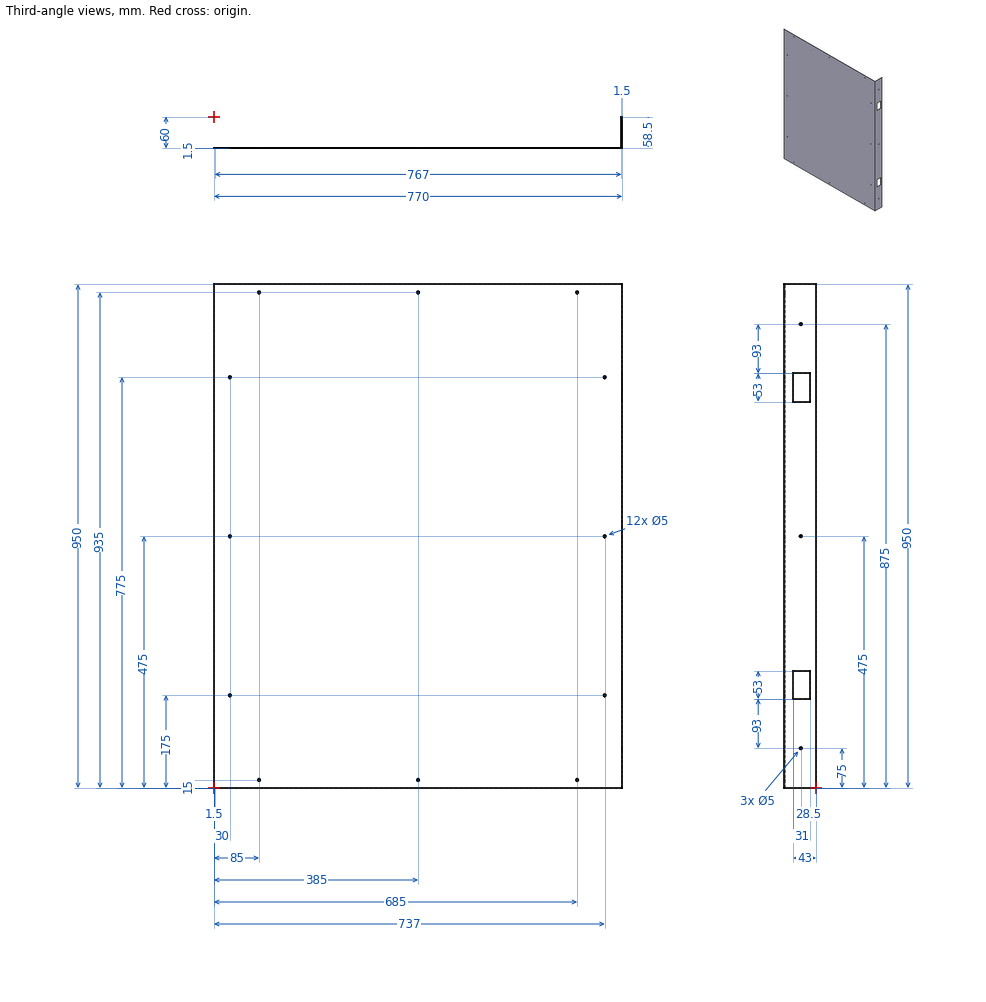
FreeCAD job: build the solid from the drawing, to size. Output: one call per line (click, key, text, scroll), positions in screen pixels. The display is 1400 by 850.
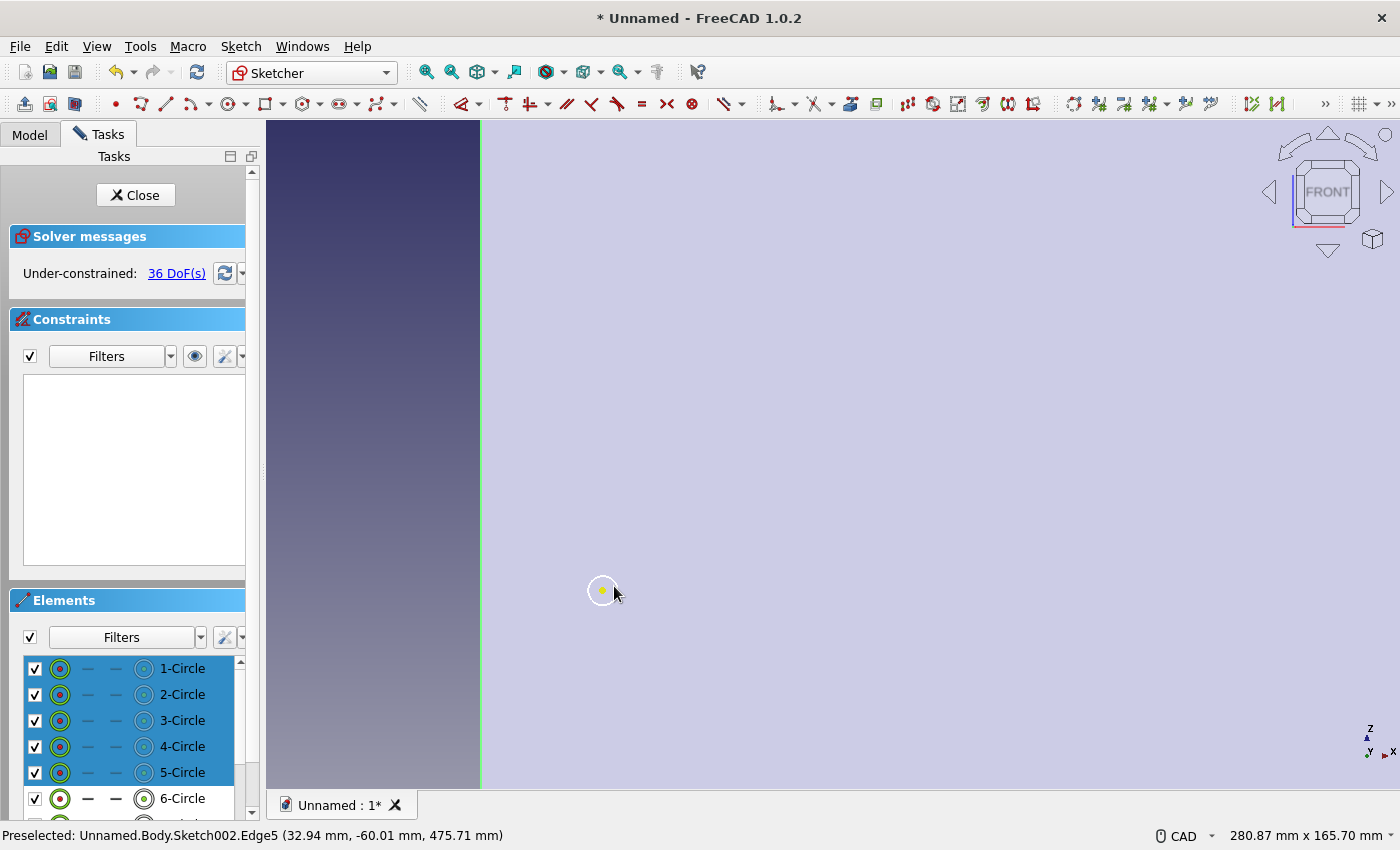
click(613, 580)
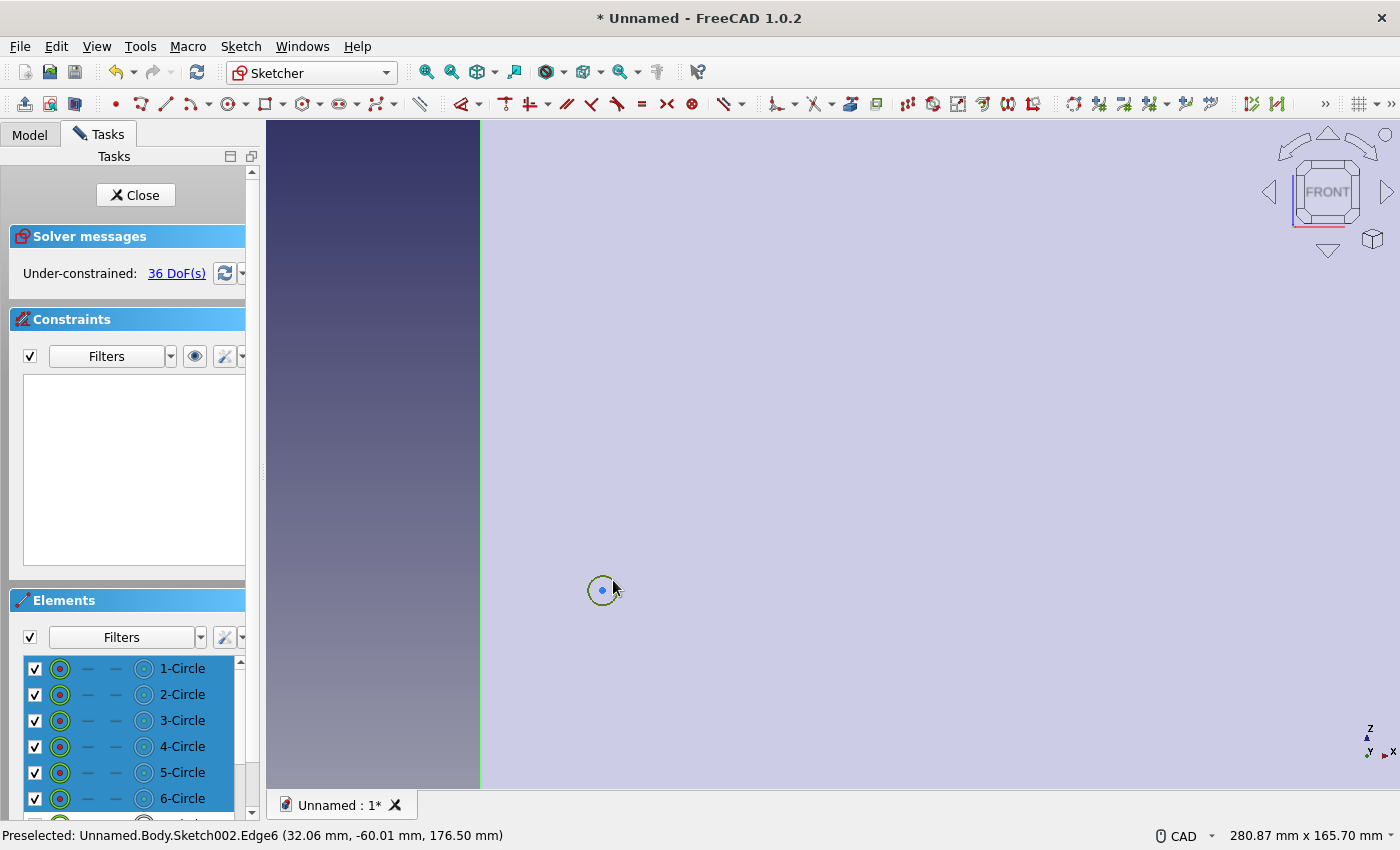
scroll(614, 586, down, 11)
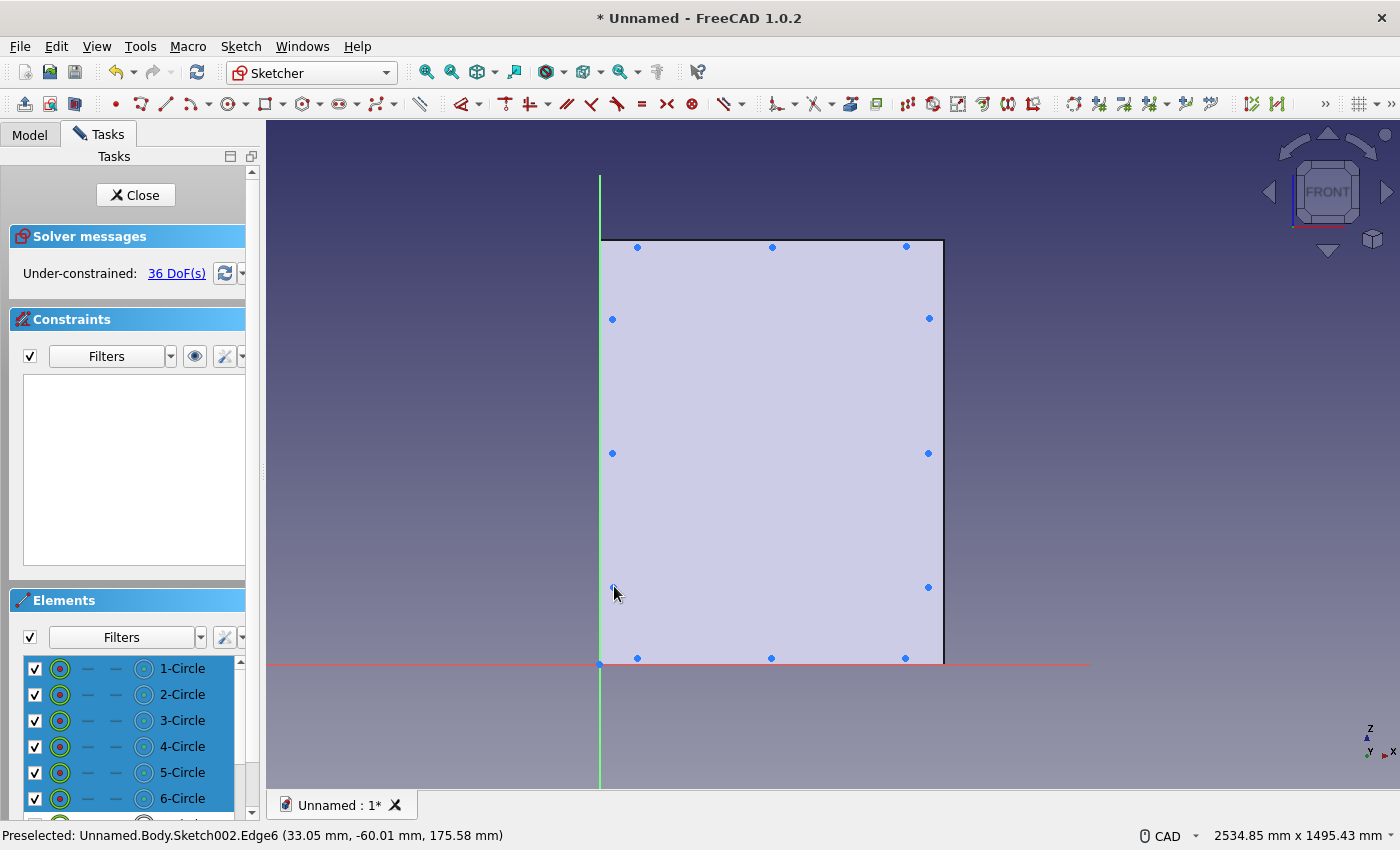
scroll(773, 246, up, 12)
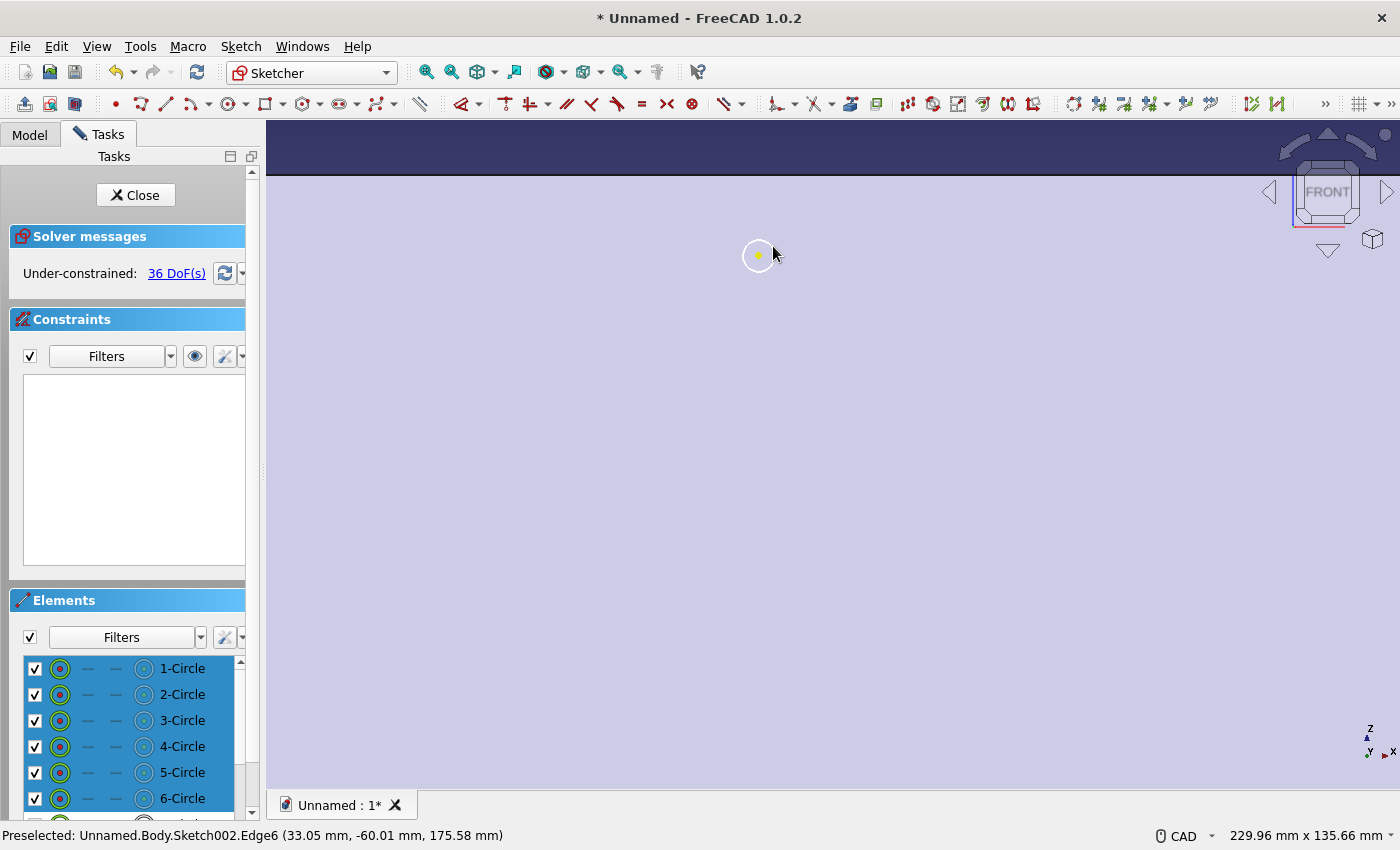
click(770, 245)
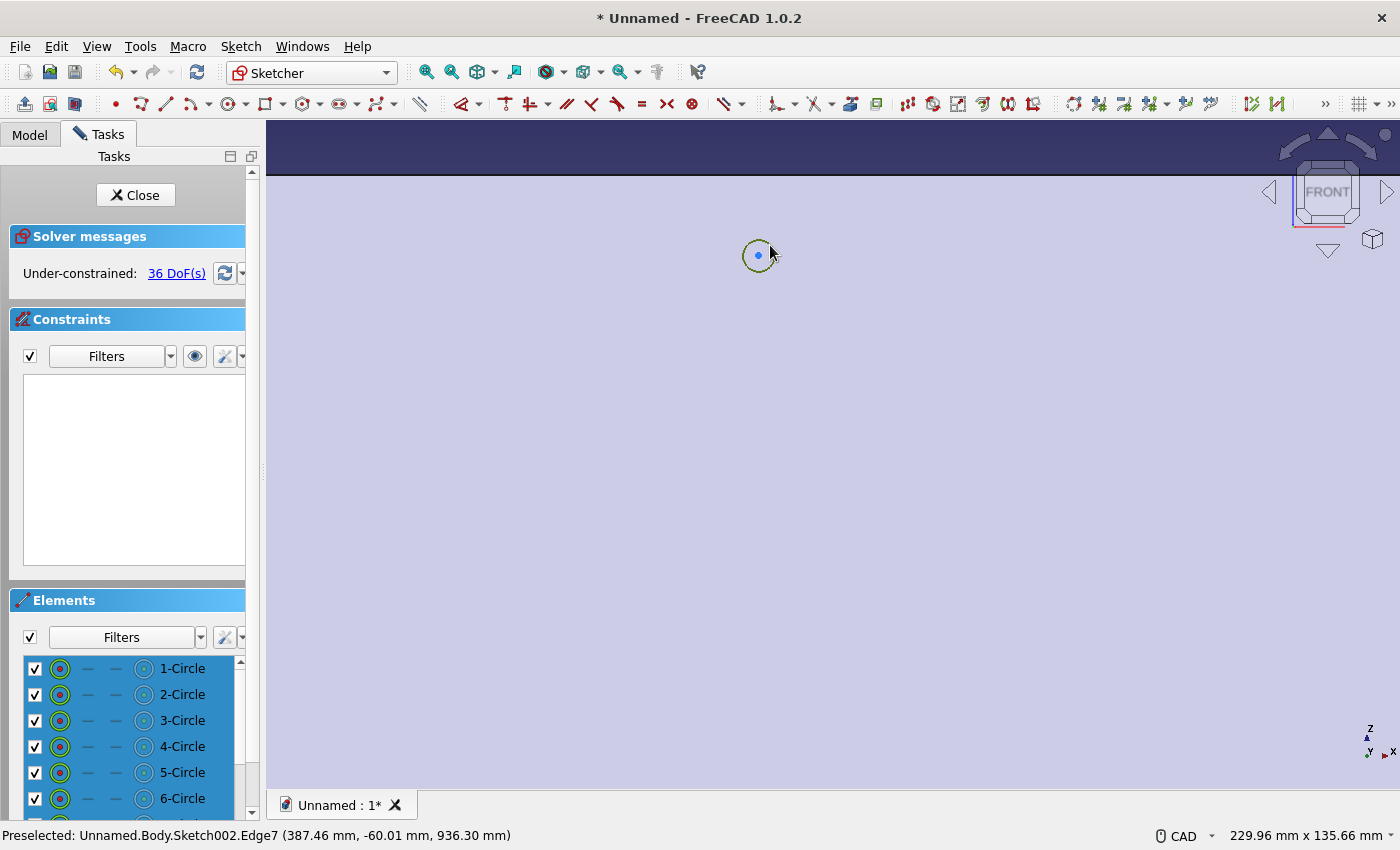
scroll(773, 246, down, 12)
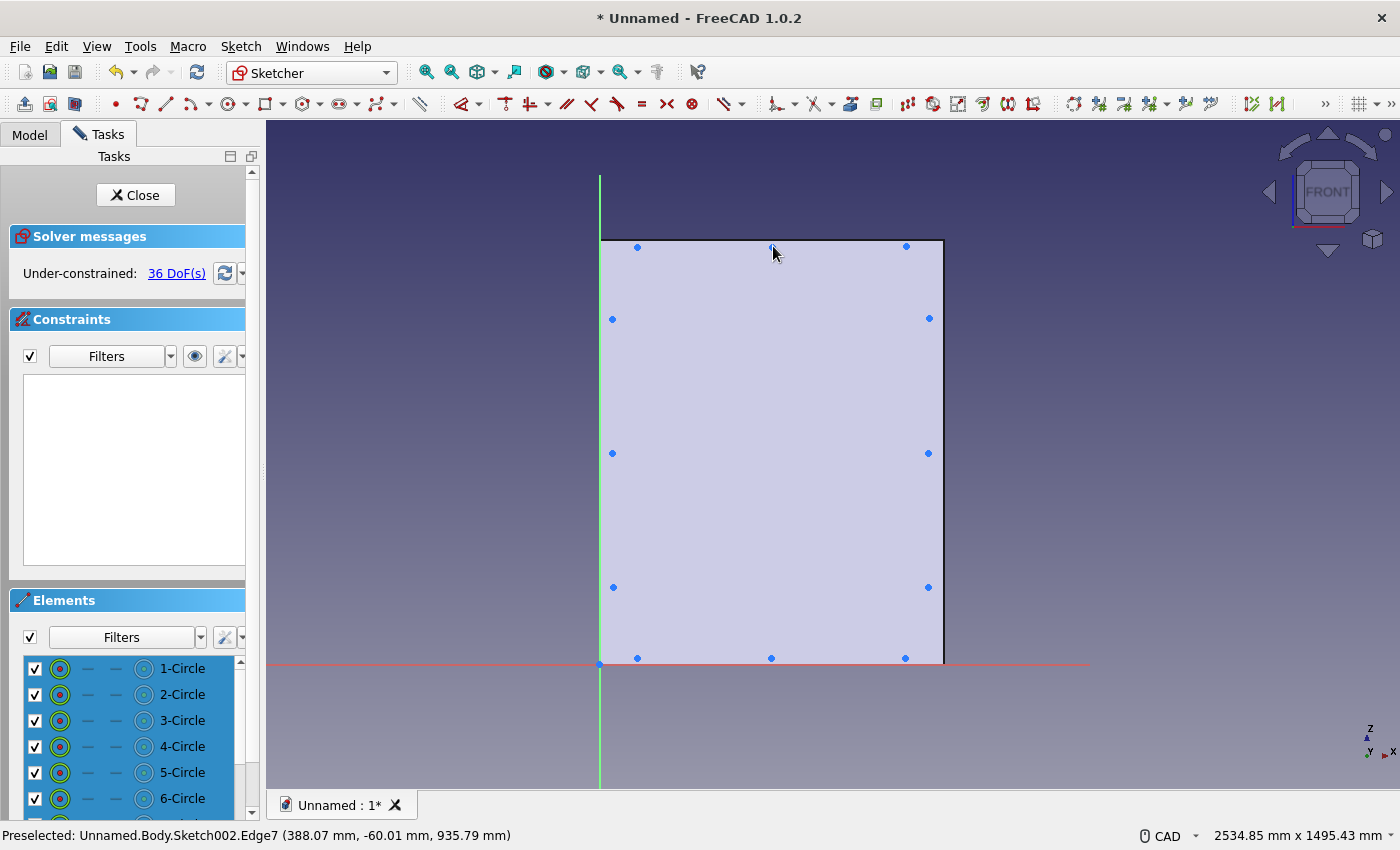
scroll(907, 246, up, 13)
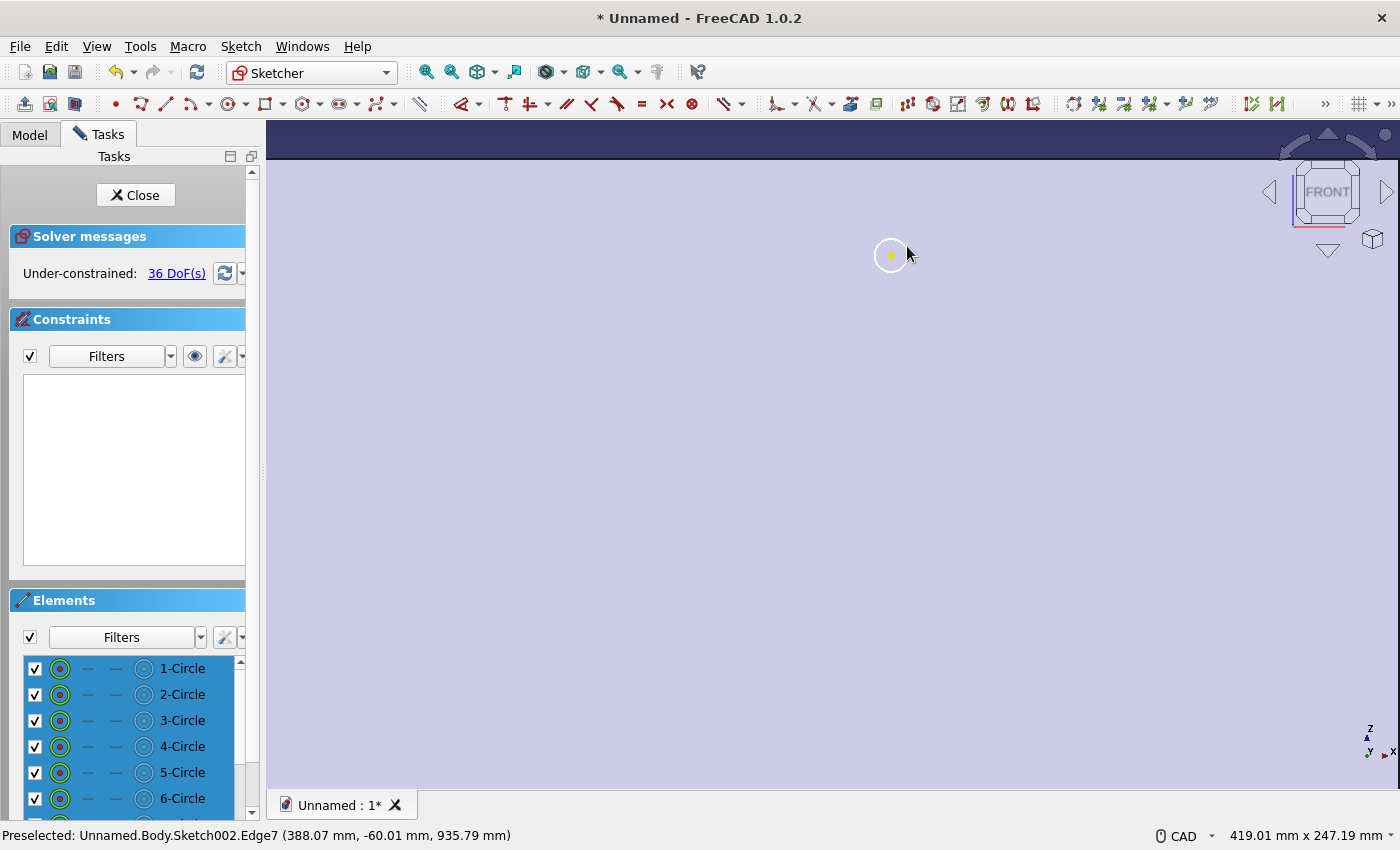
click(903, 244)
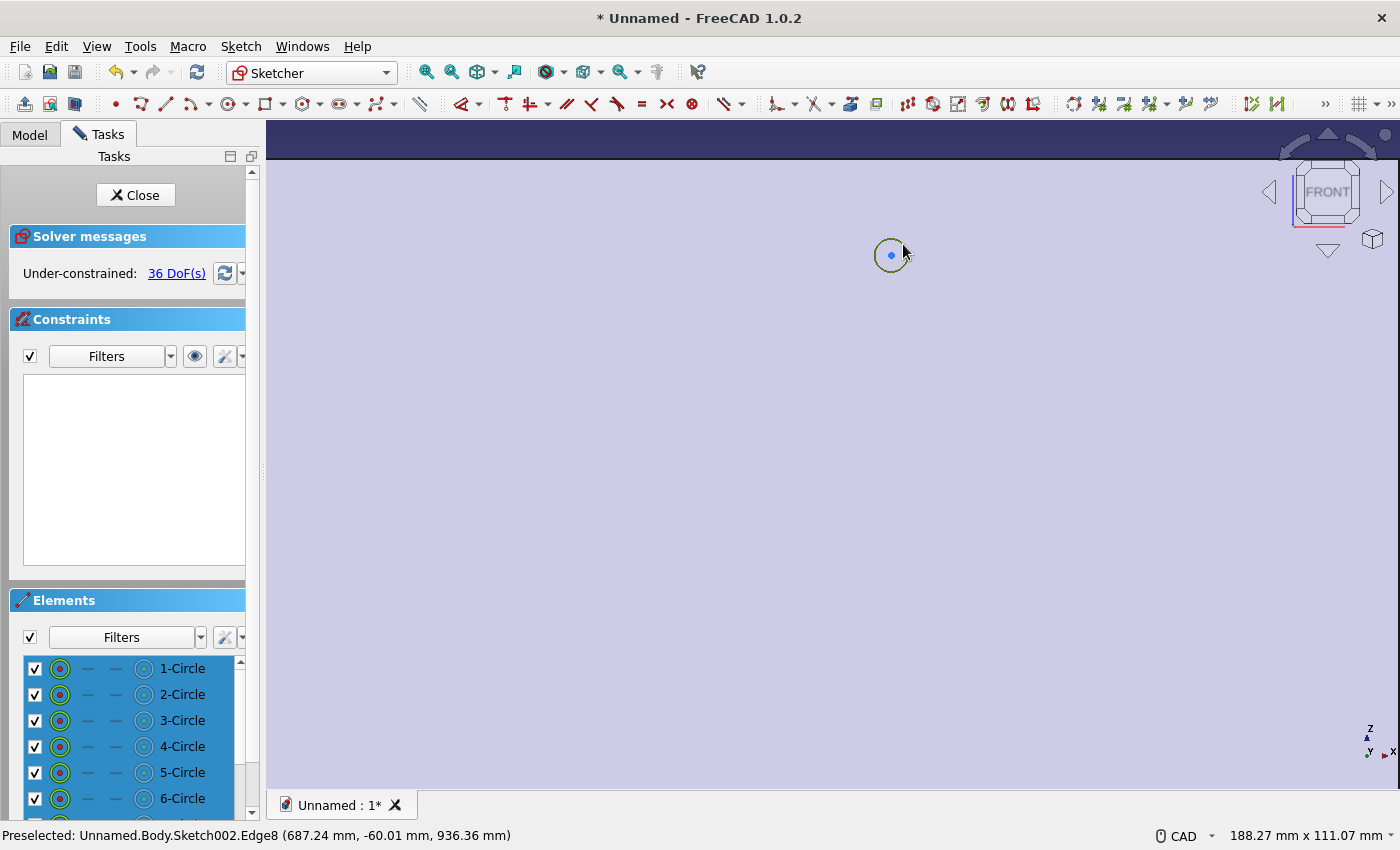
scroll(907, 246, down, 13)